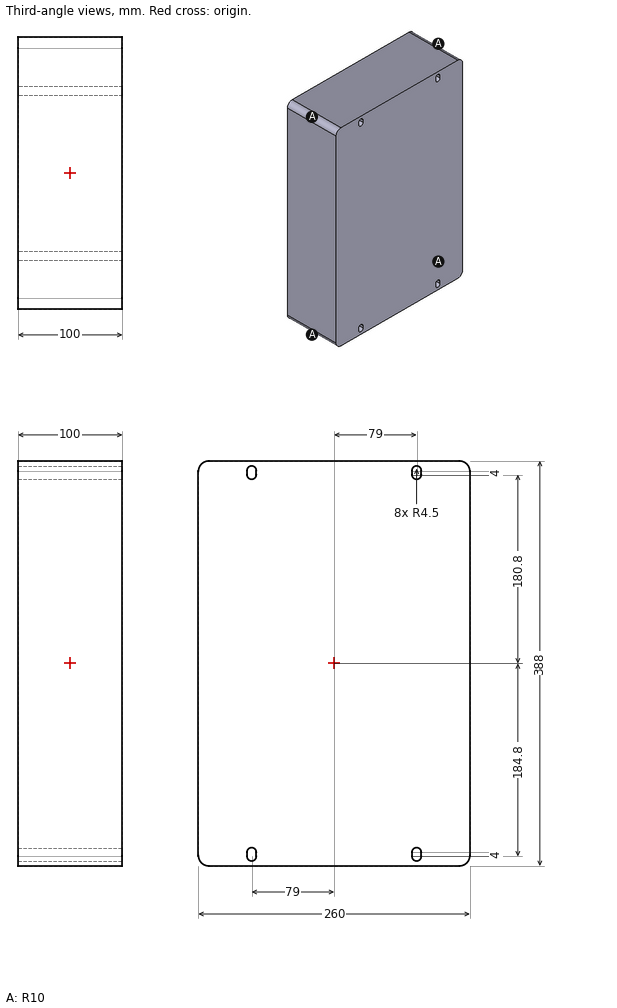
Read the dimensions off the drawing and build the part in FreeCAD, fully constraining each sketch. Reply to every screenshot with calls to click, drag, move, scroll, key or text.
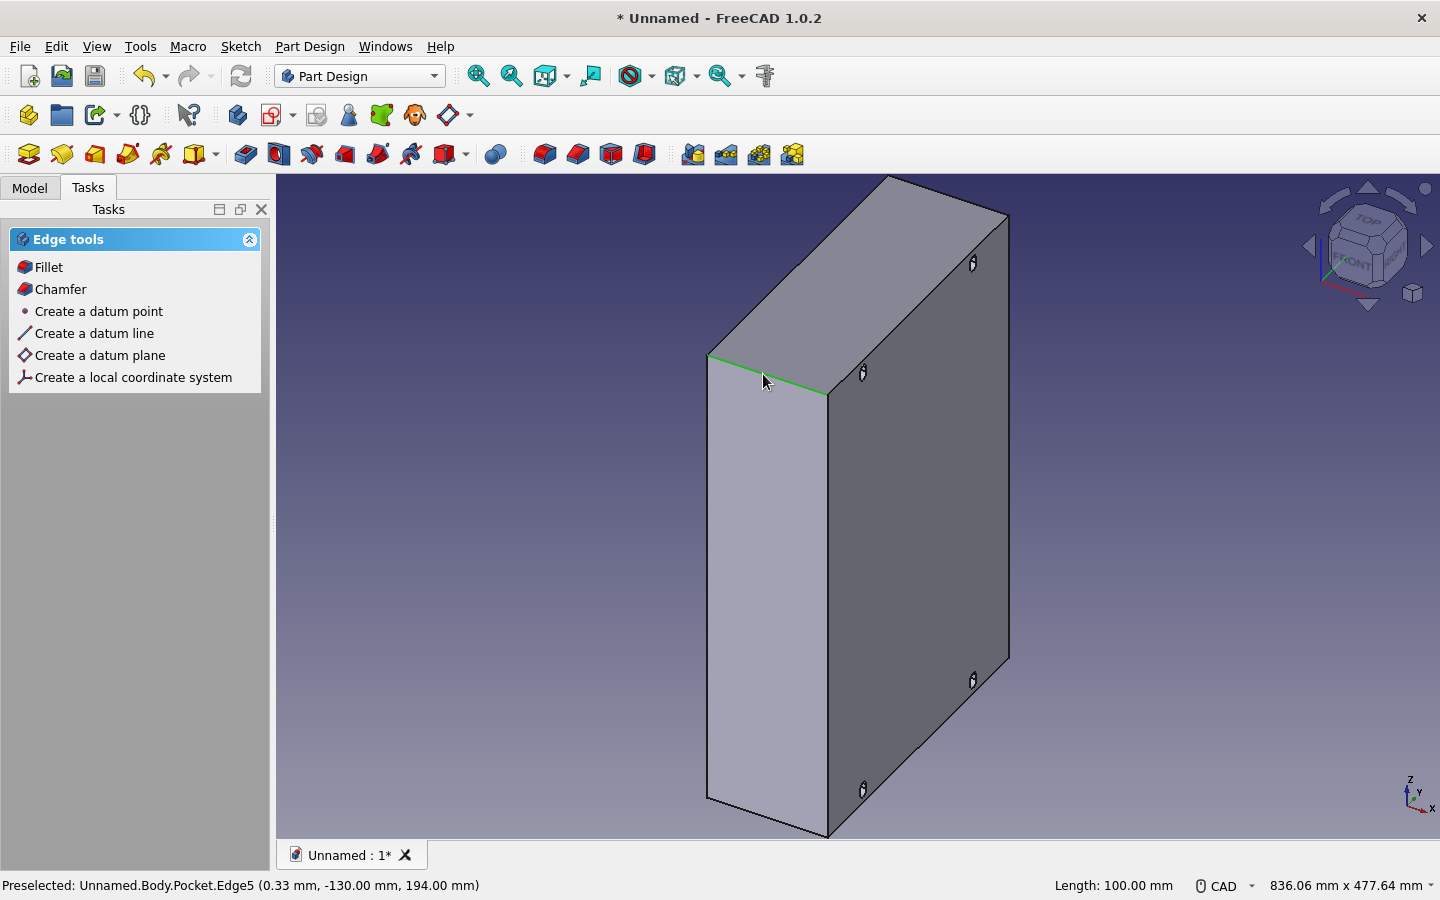
key(0)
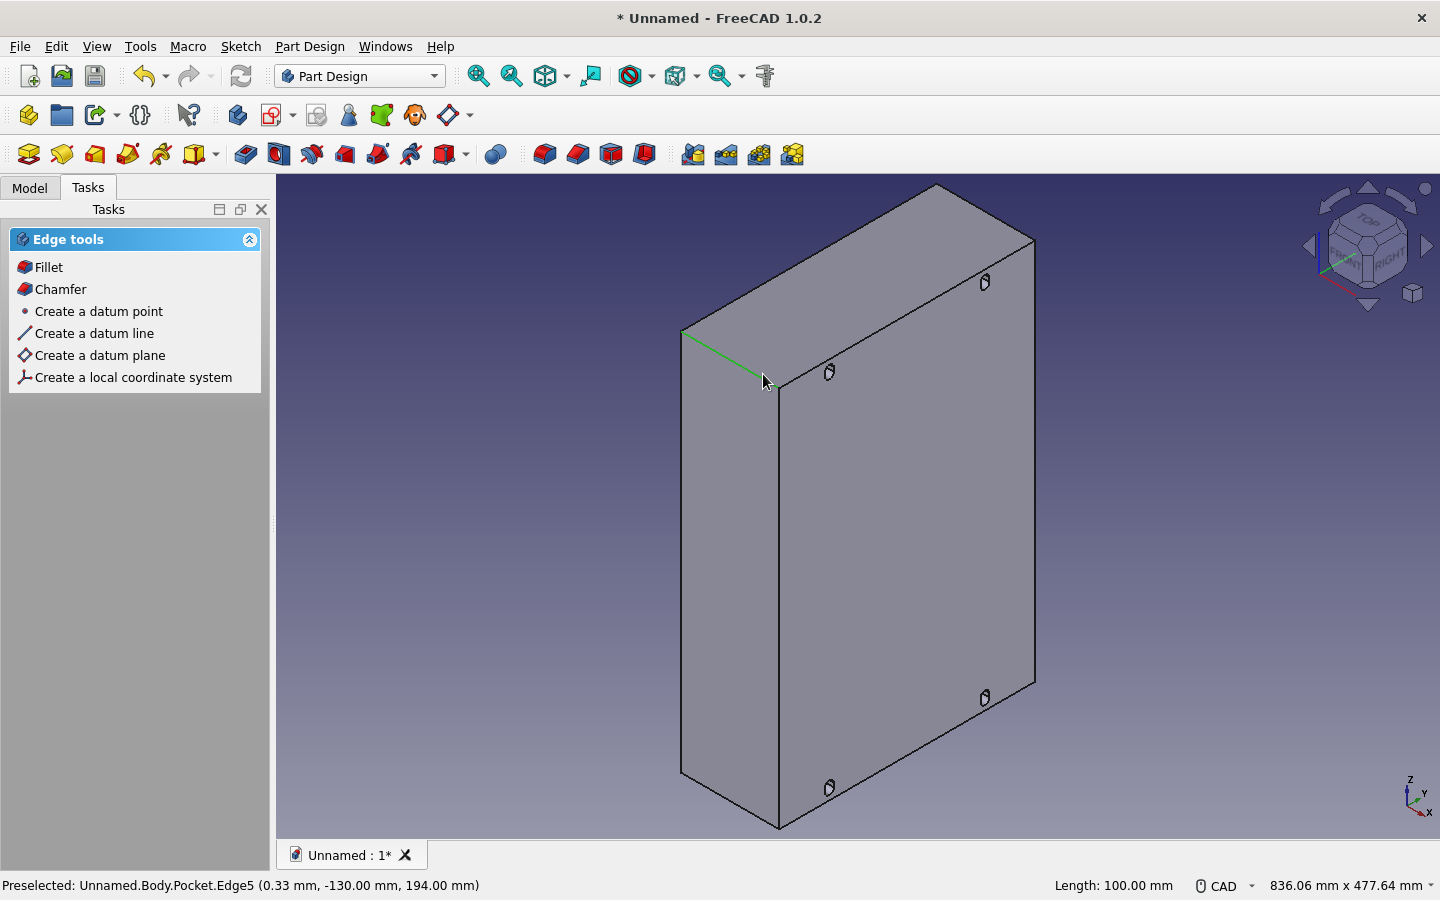
key(2)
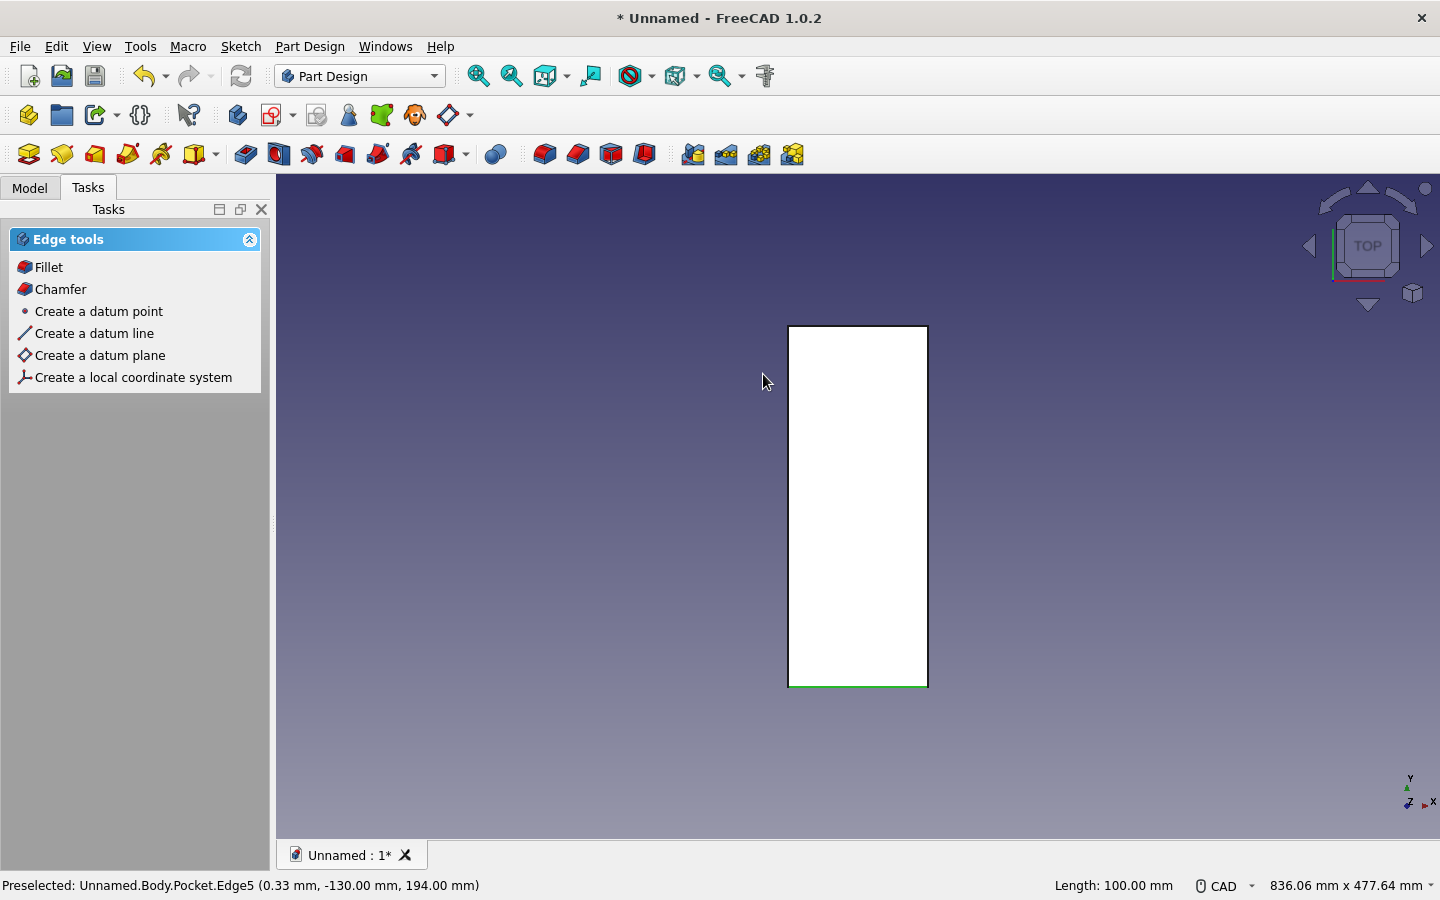
click(858, 325, ctrl)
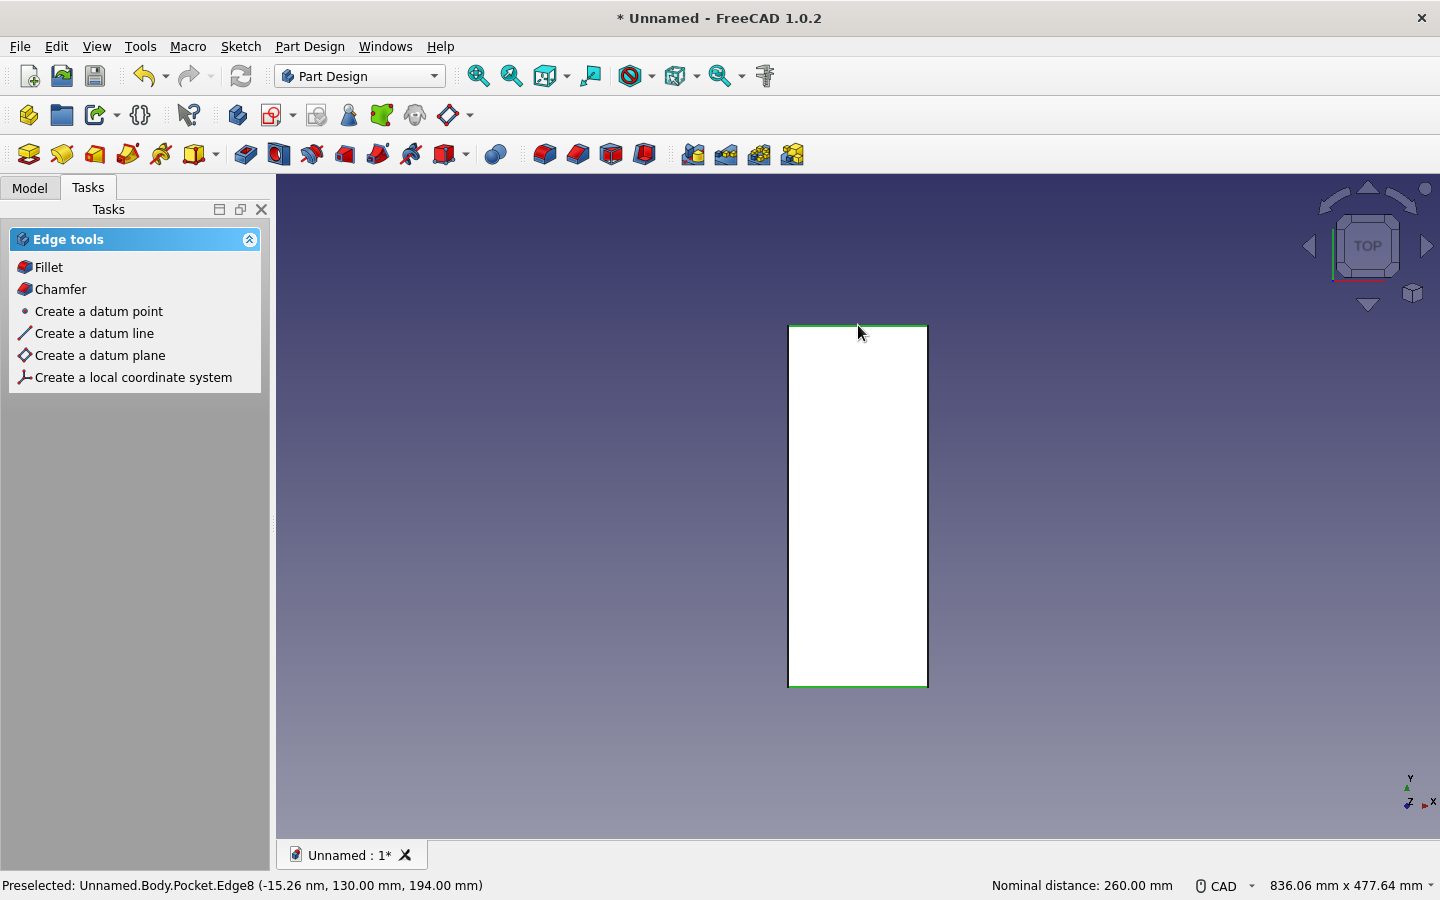
key(1)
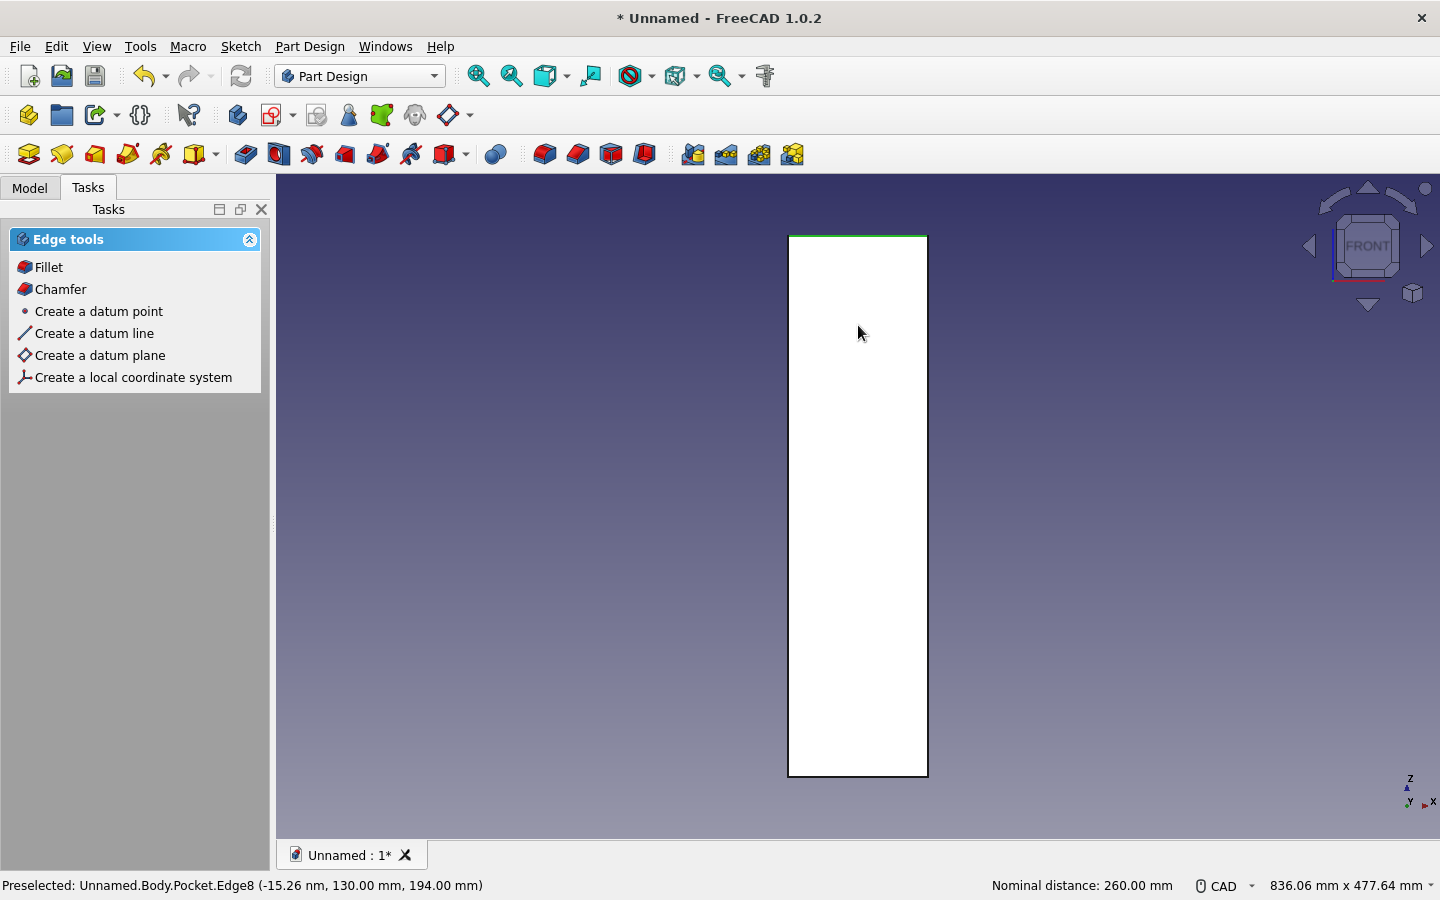
click(858, 776, ctrl)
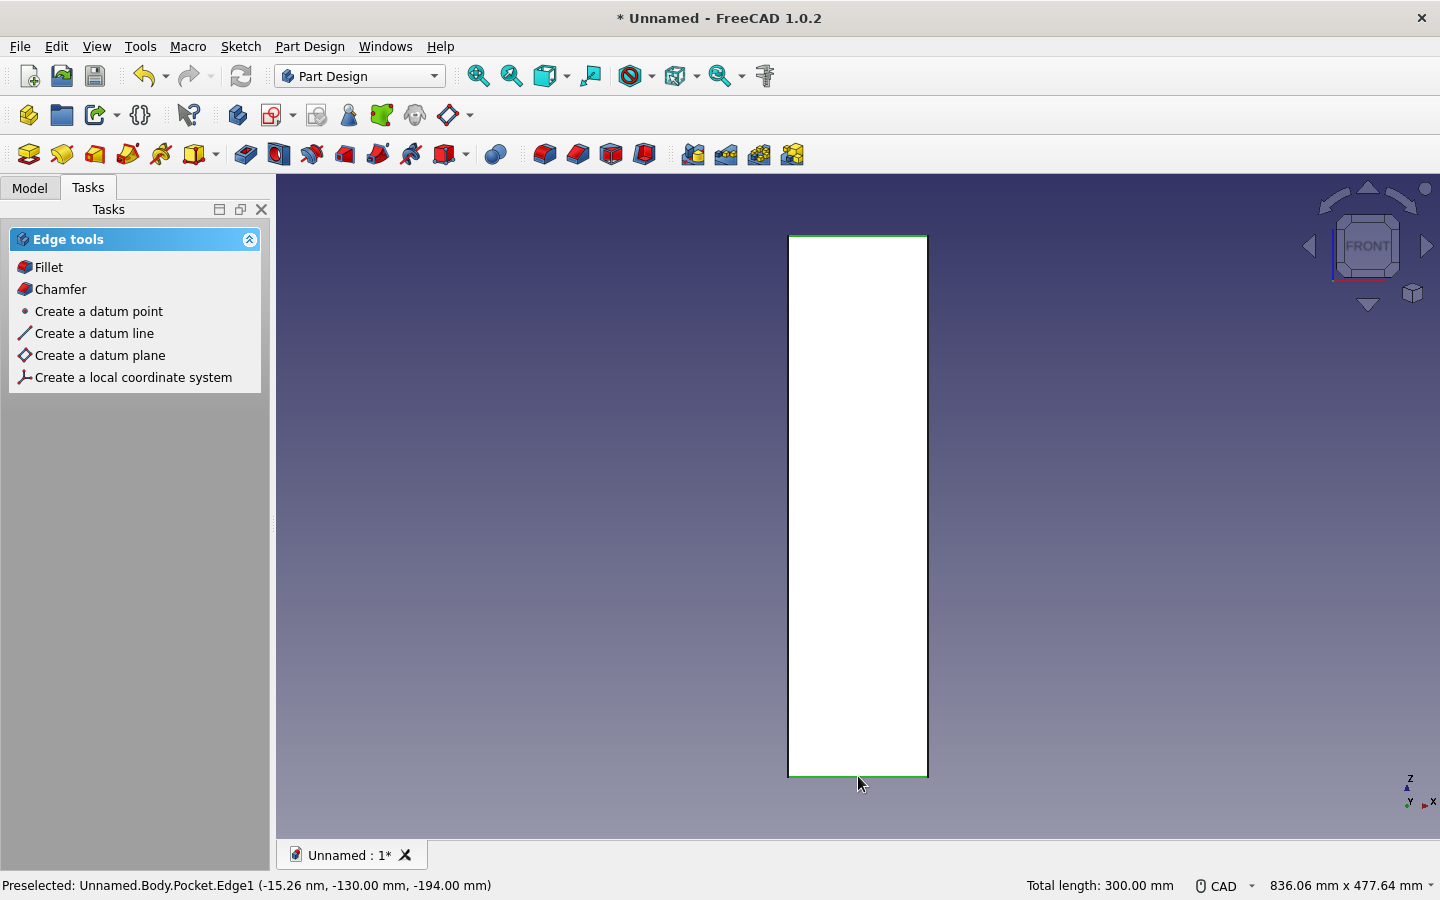
key(3)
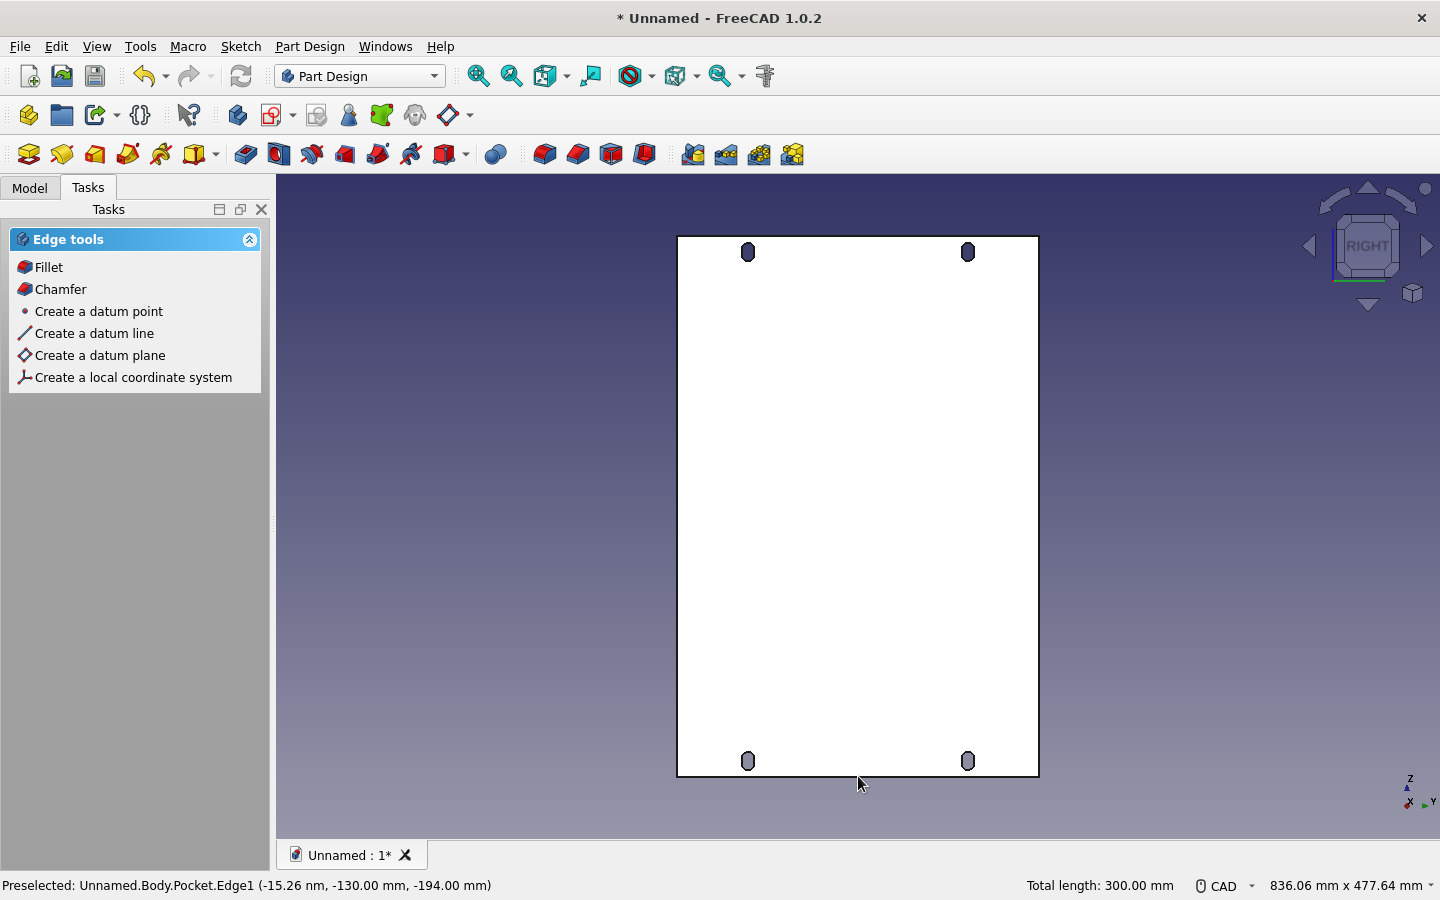
key(5)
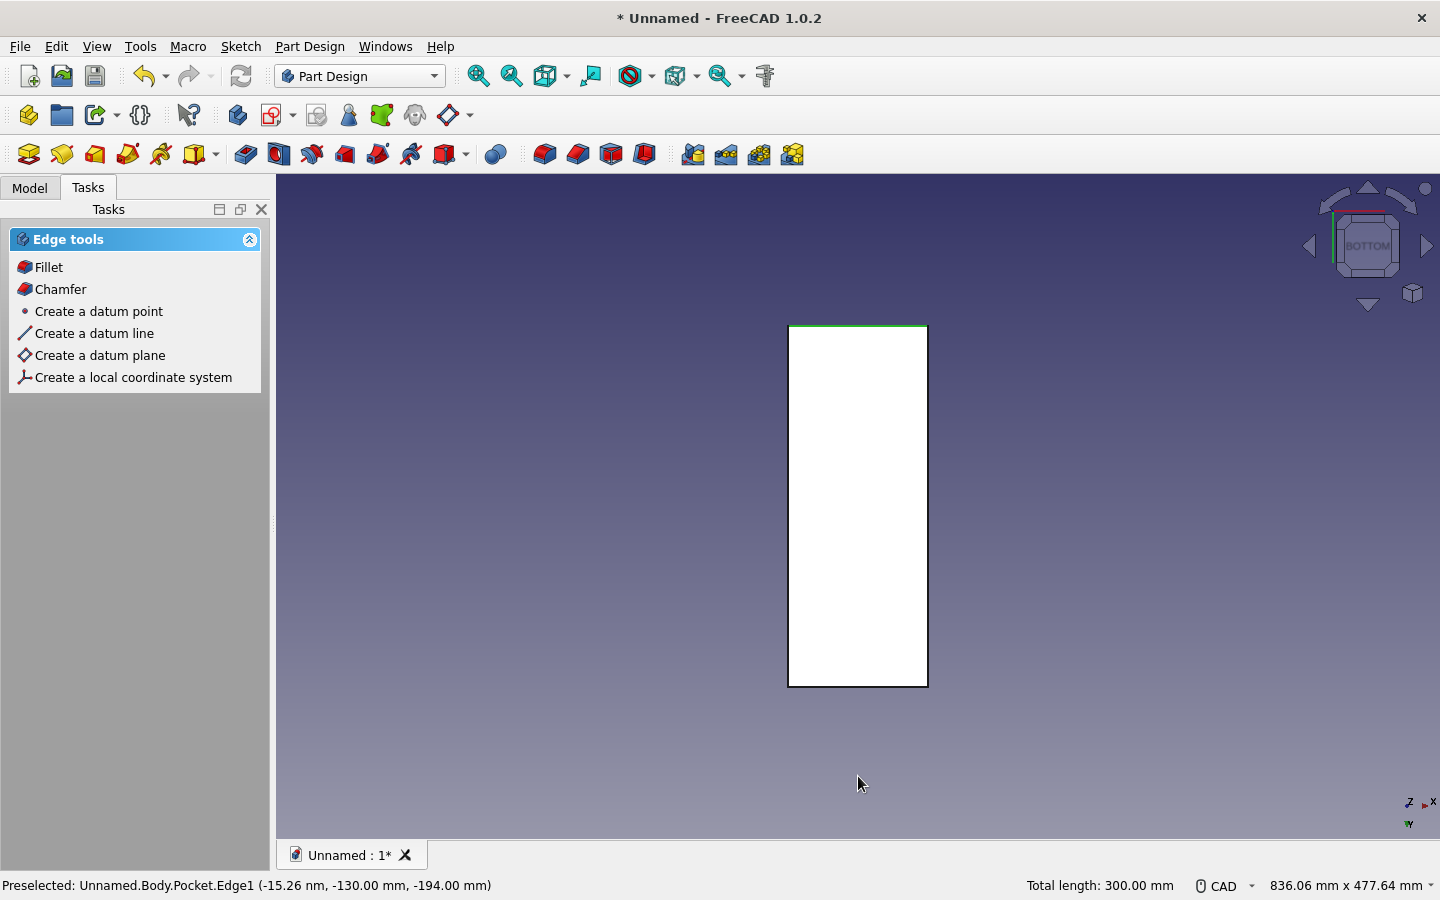
click(858, 686, ctrl)